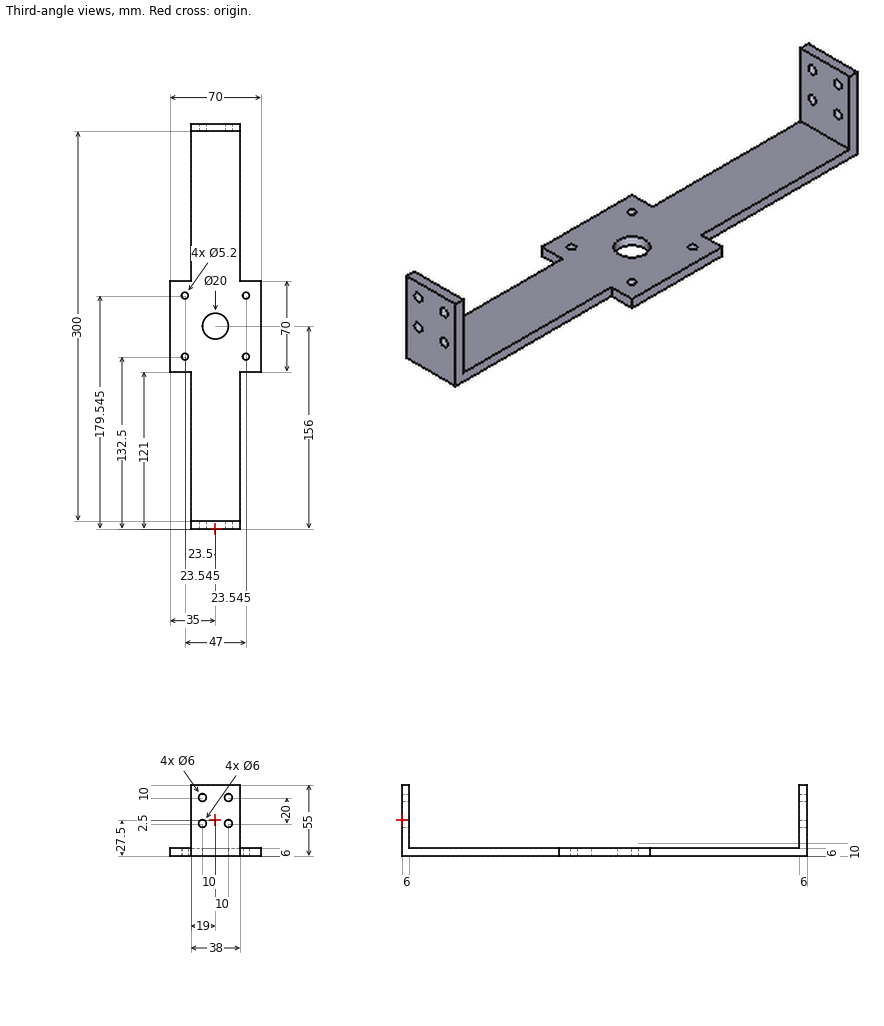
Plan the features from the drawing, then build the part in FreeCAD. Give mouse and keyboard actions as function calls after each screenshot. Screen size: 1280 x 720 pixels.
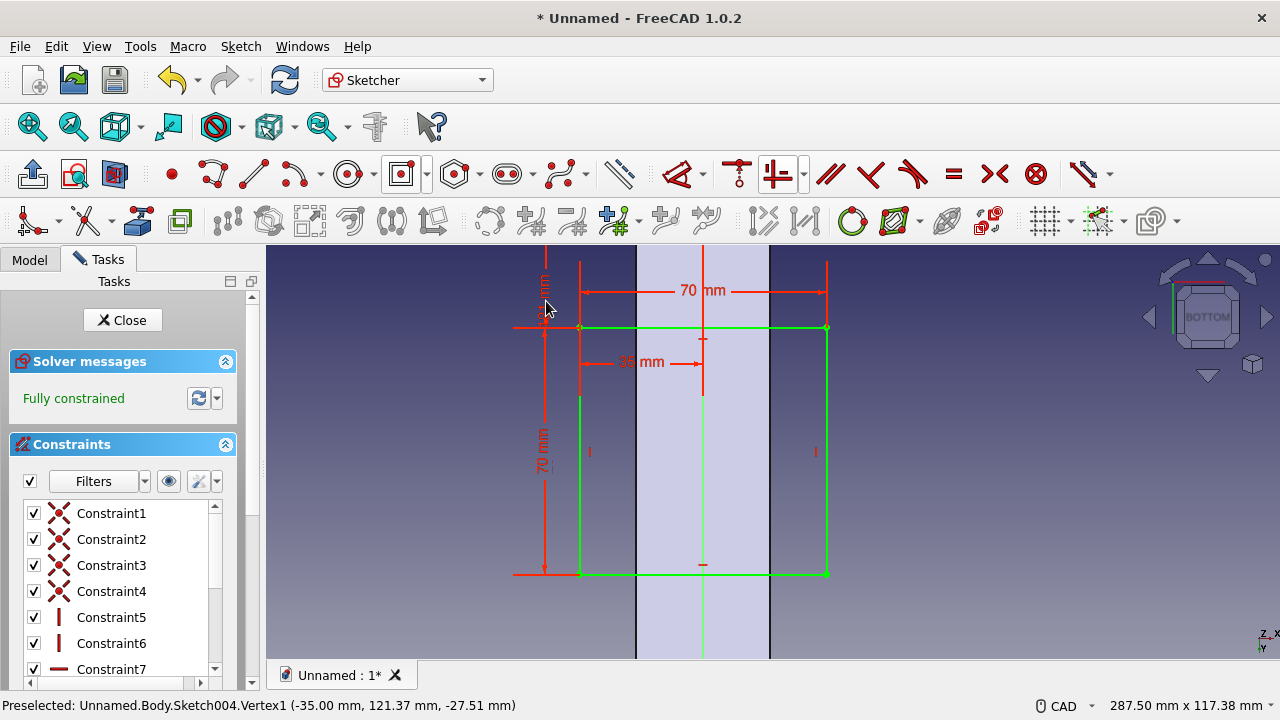
click(123, 320)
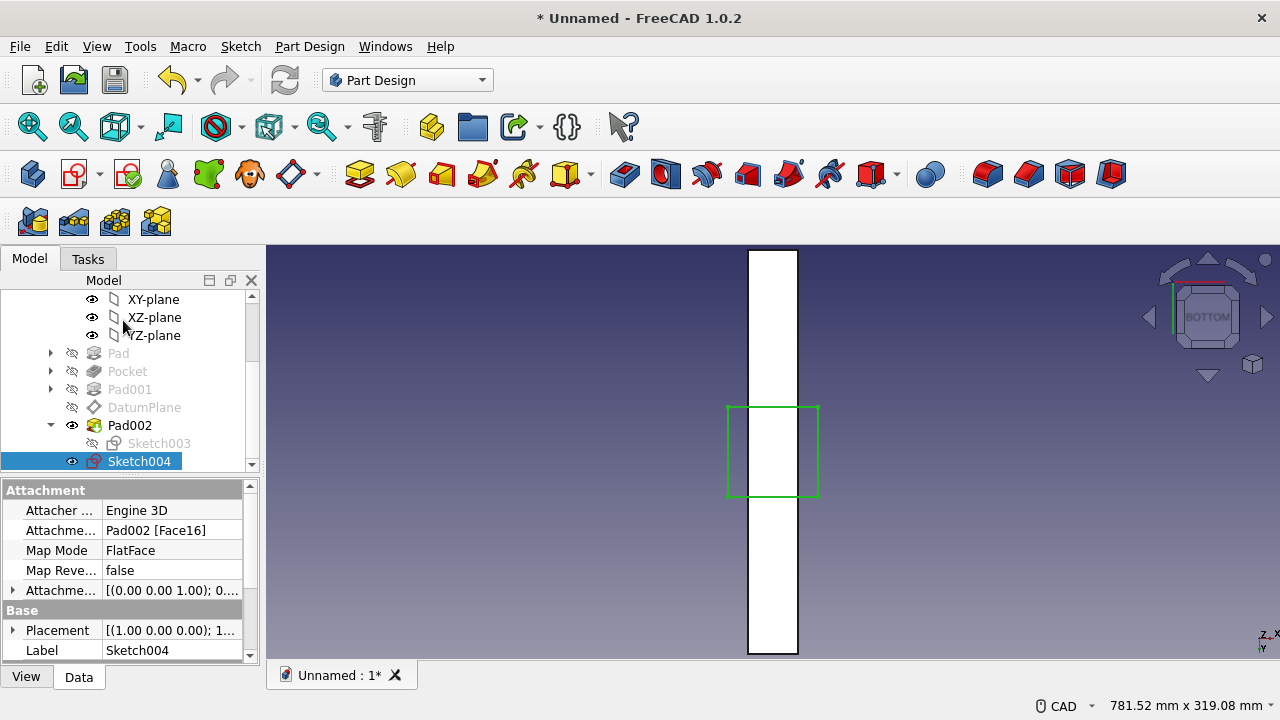
click(360, 174)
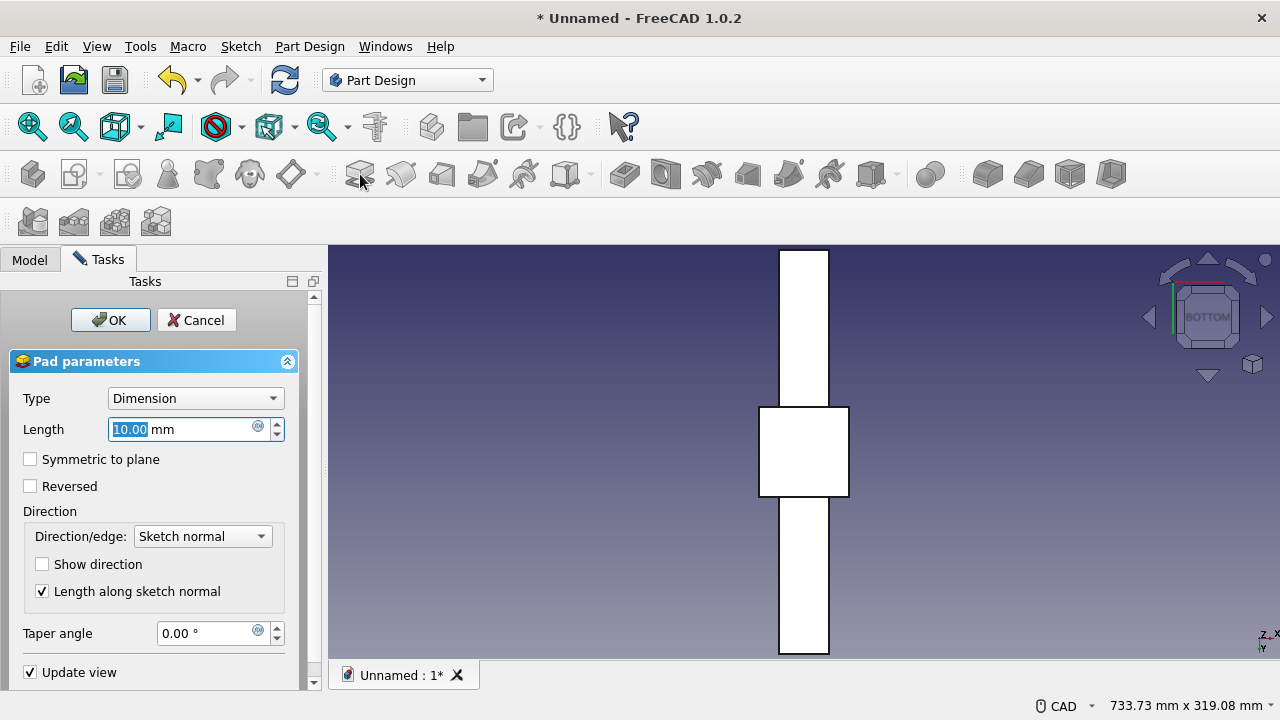
text(6)
key(Tab)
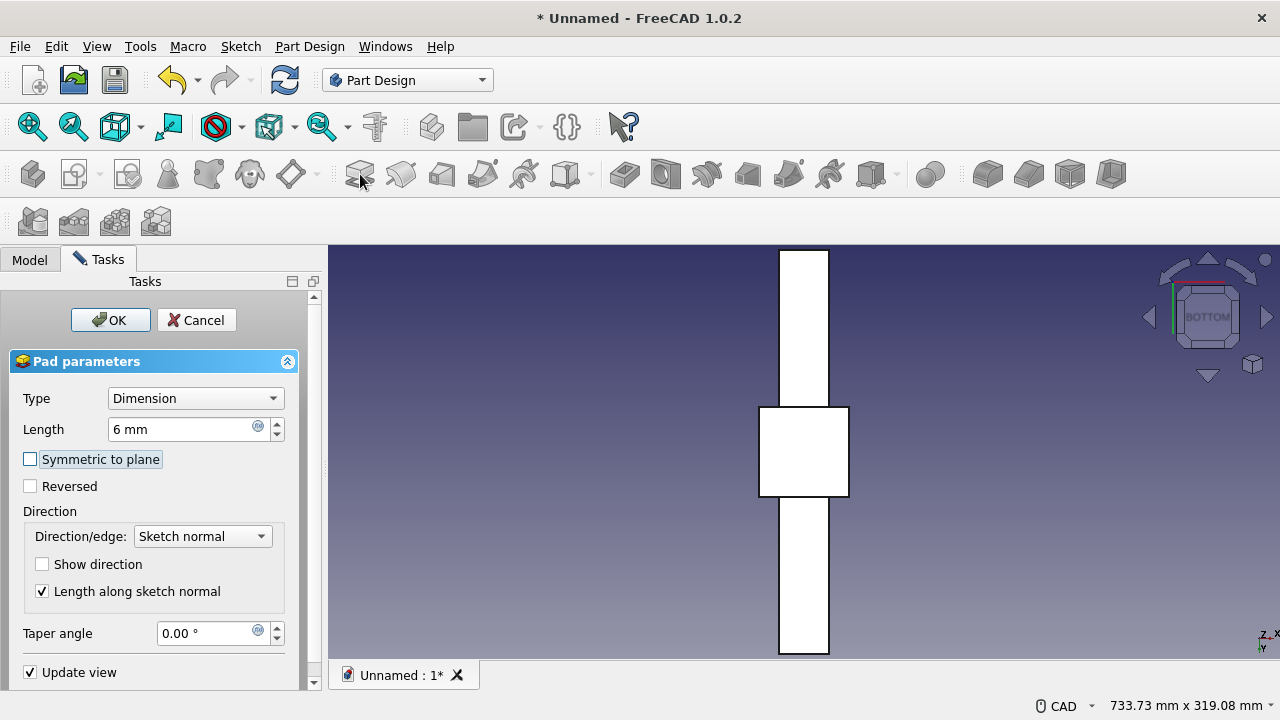
click(31, 486)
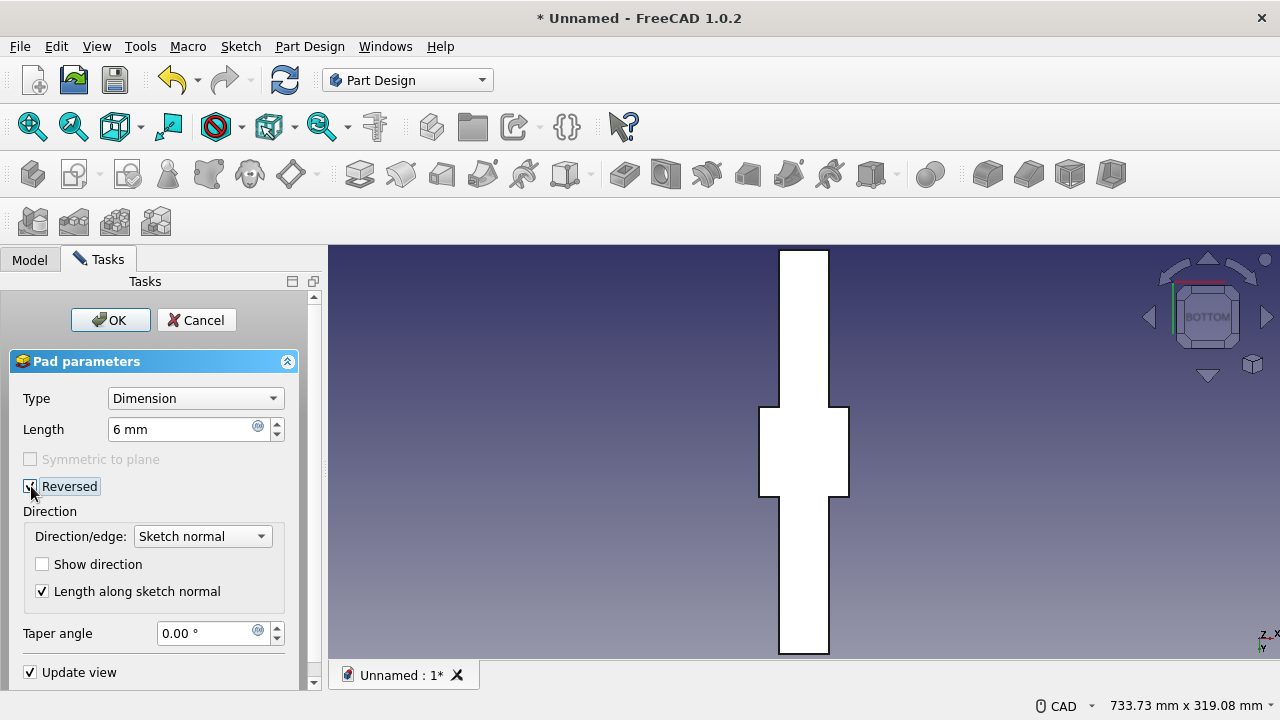
click(111, 320)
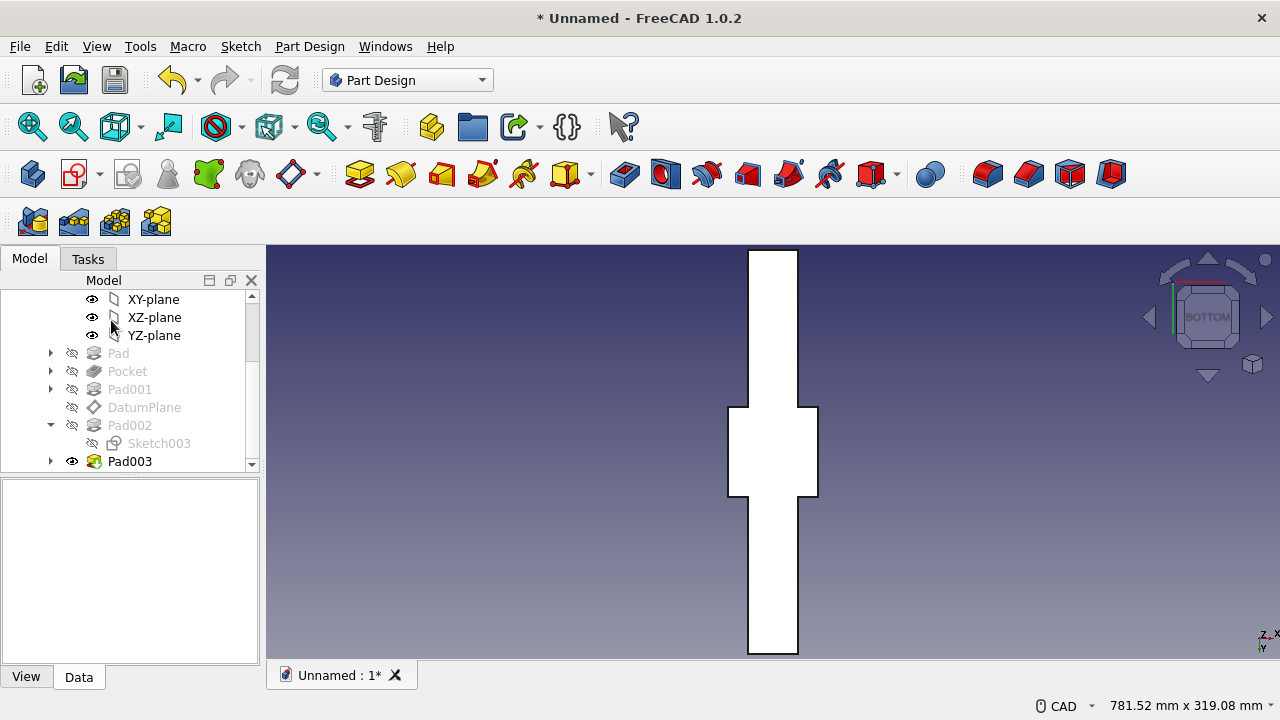
click(773, 451)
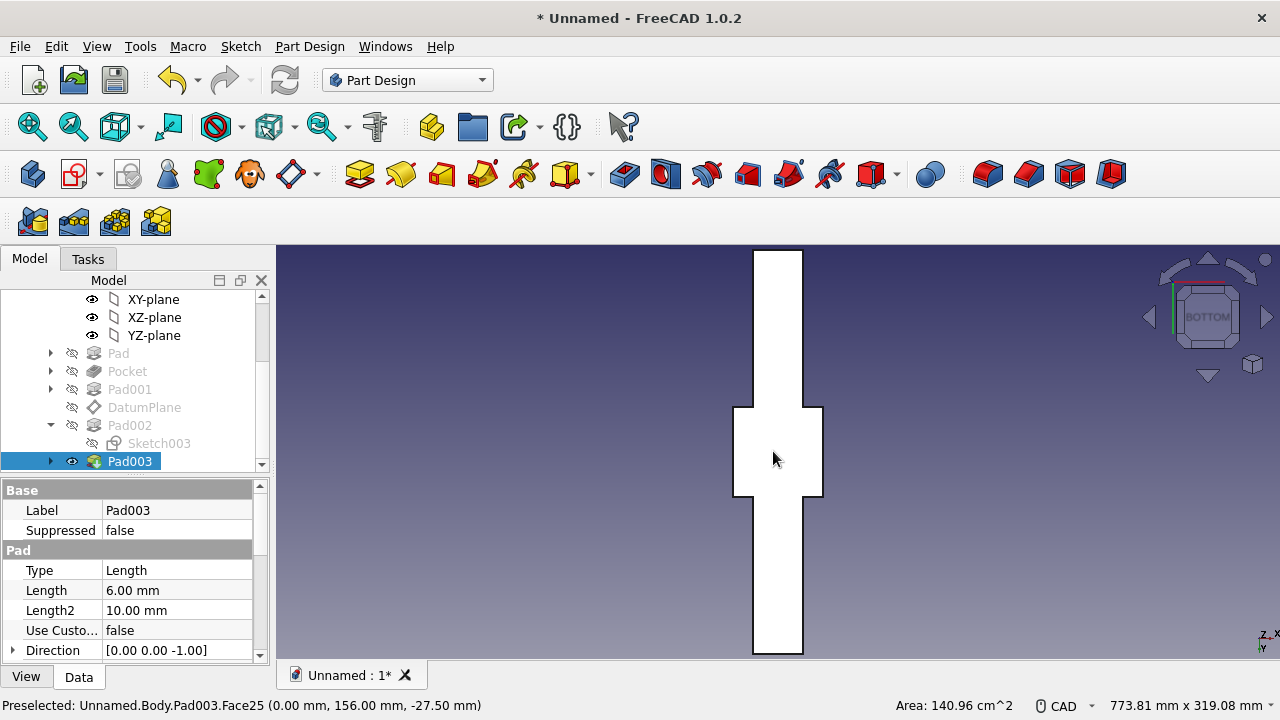
click(74, 174)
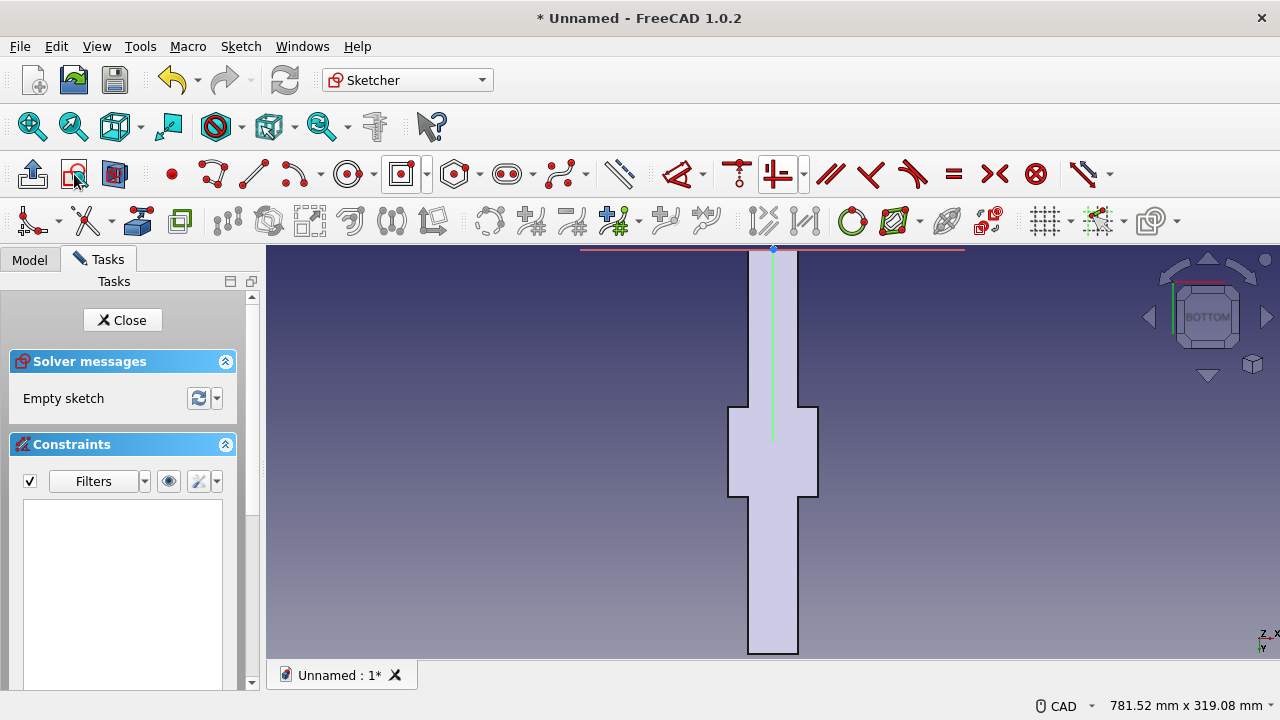
scroll(795, 452, up, 7)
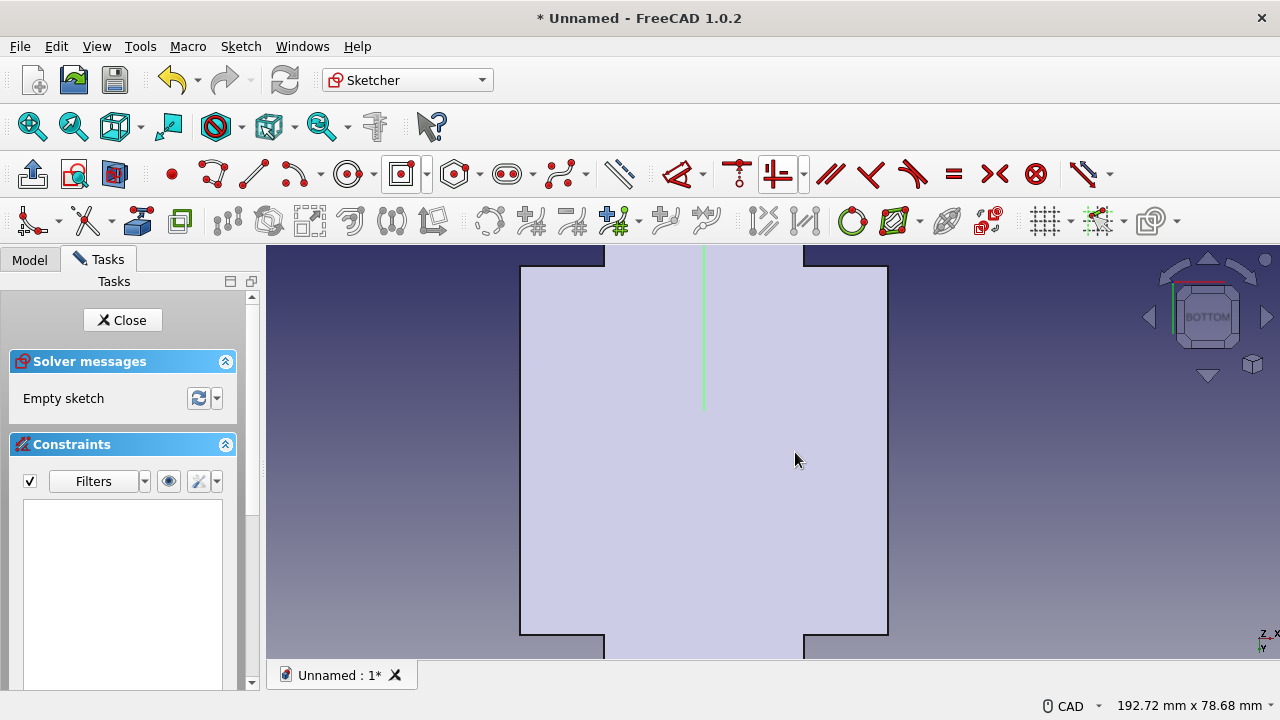
click(348, 174)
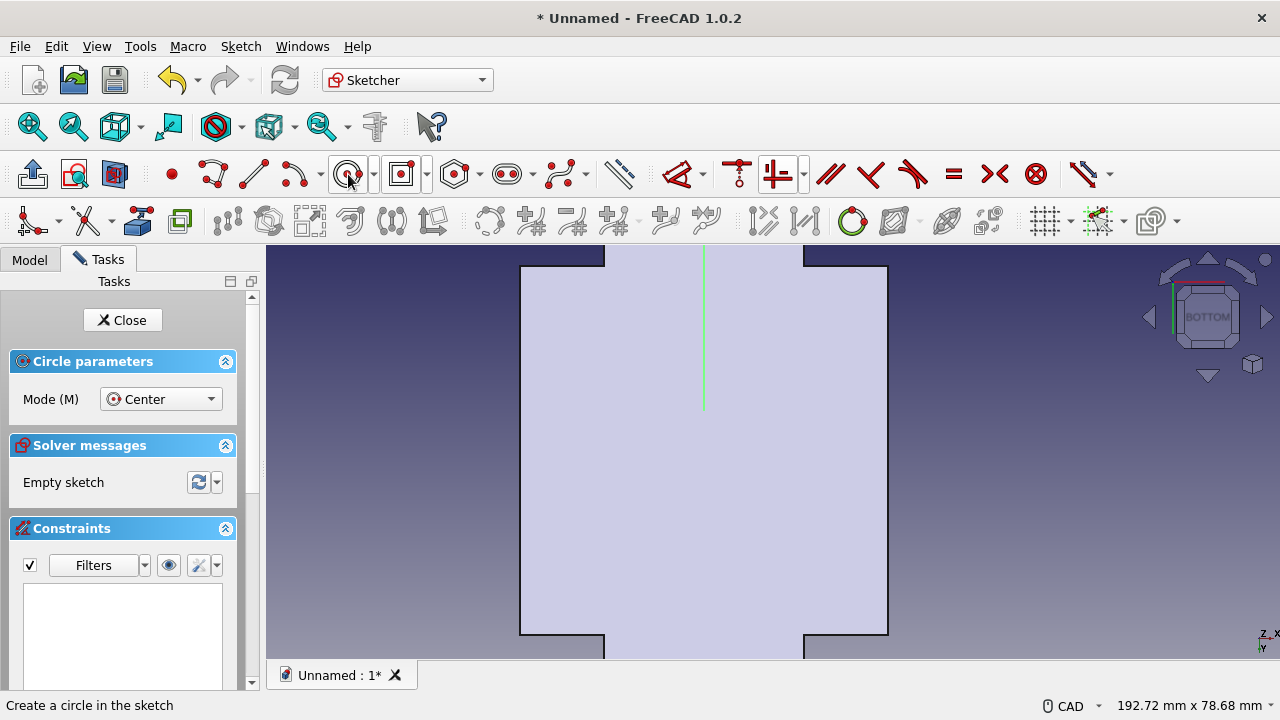
scroll(580, 574, up, 3)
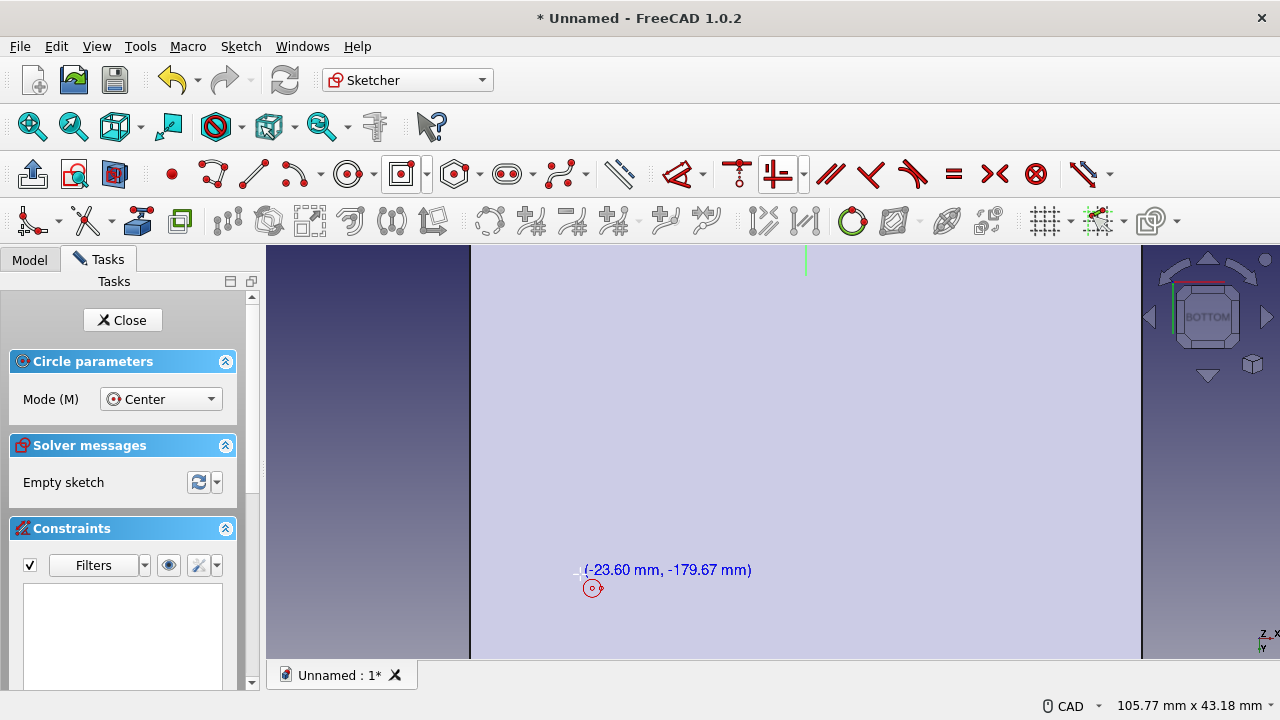
click(580, 574)
move(598, 556)